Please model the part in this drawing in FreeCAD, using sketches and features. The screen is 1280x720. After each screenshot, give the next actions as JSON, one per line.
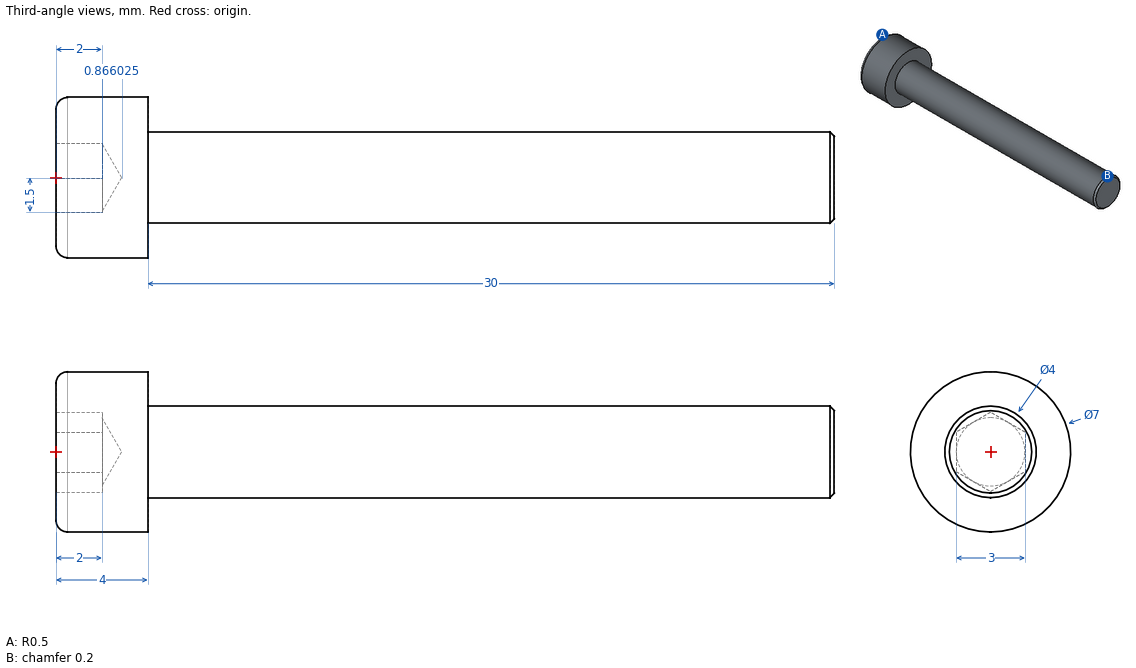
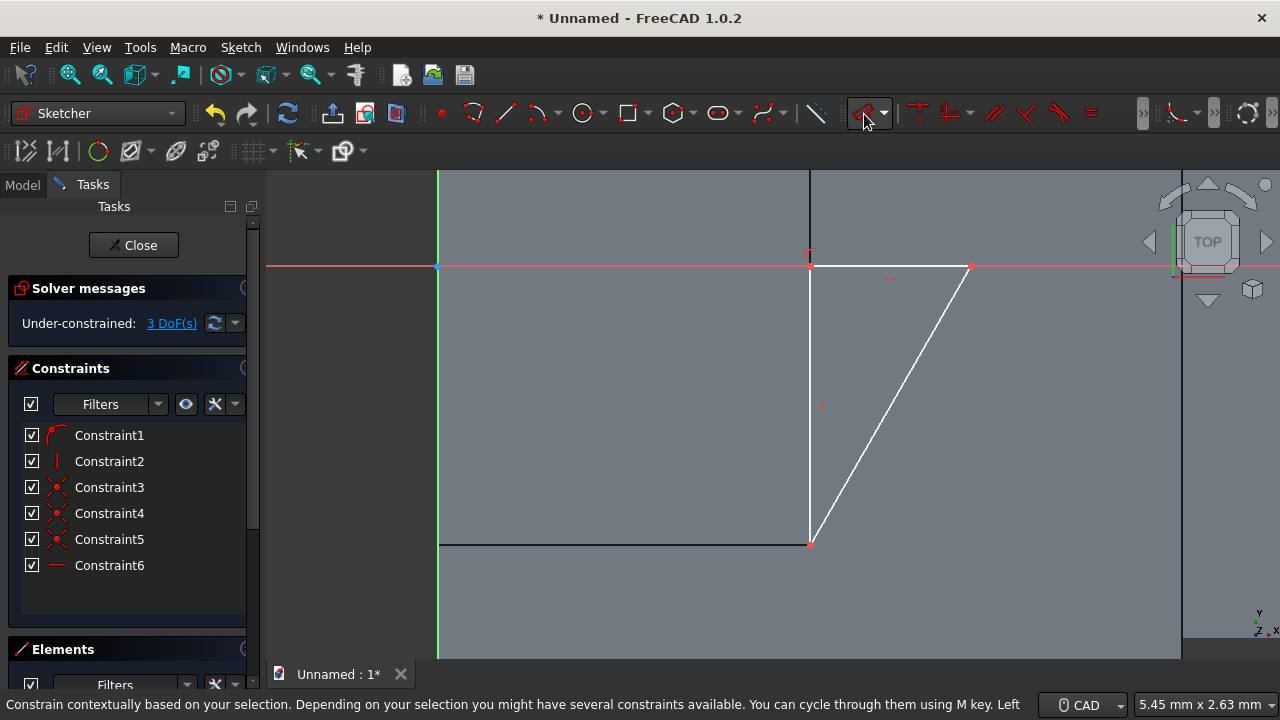
{"action": "left_click", "coordinate": [810, 266]}
{"action": "left_click", "coordinate": [624, 232]}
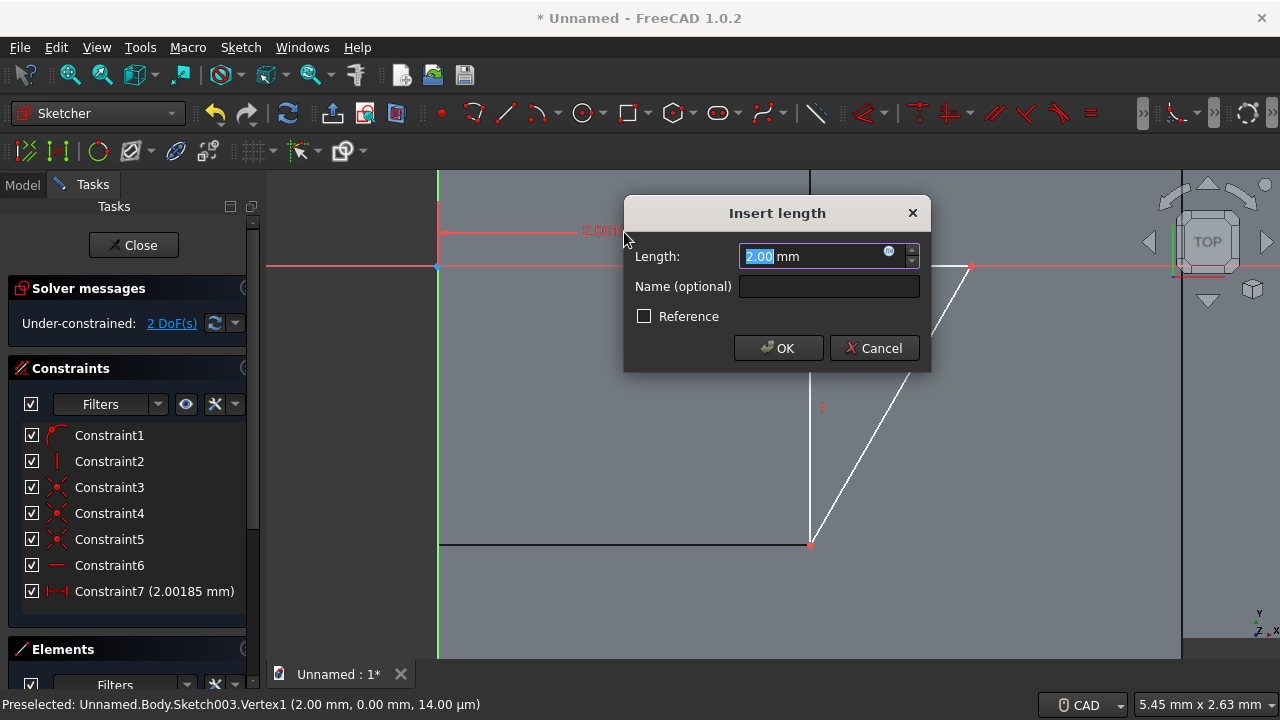
{"action": "type", "text": "2"}
{"action": "key", "text": "Return"}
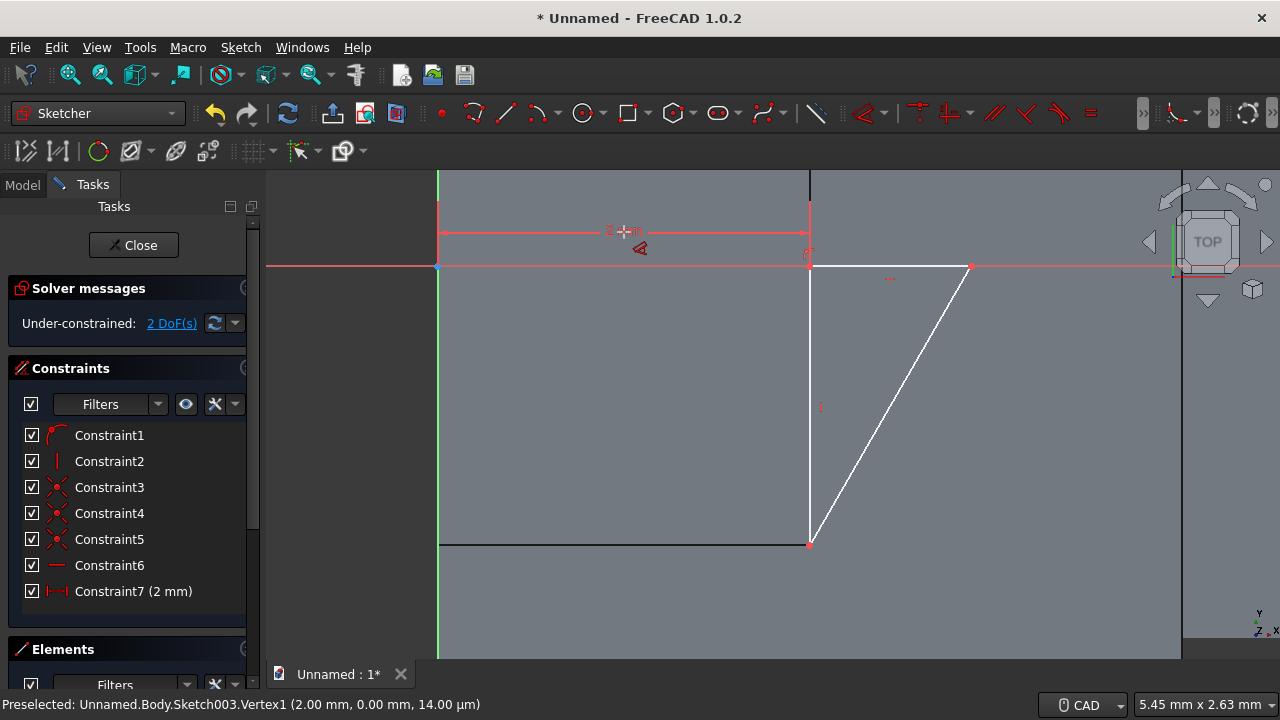
{"action": "left_click", "coordinate": [810, 350]}
{"action": "left_click", "coordinate": [844, 406]}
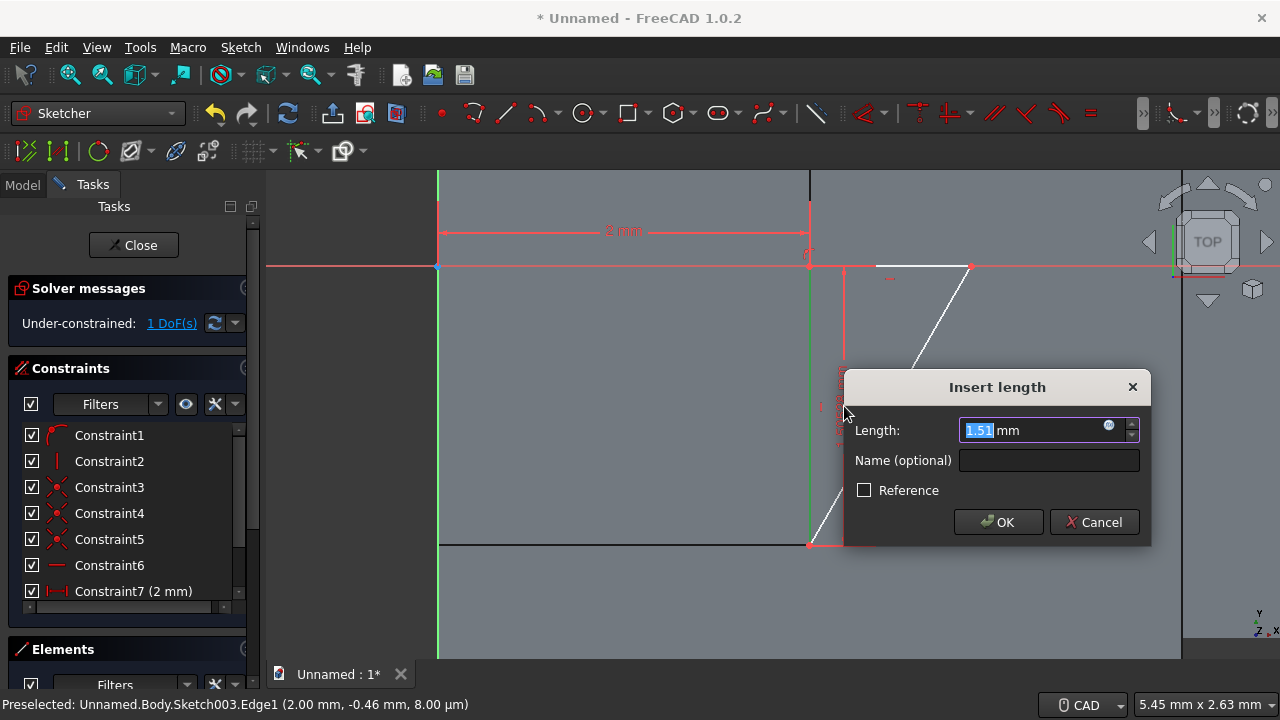
{"action": "type", "text": "1.5"}
{"action": "key", "text": "Return"}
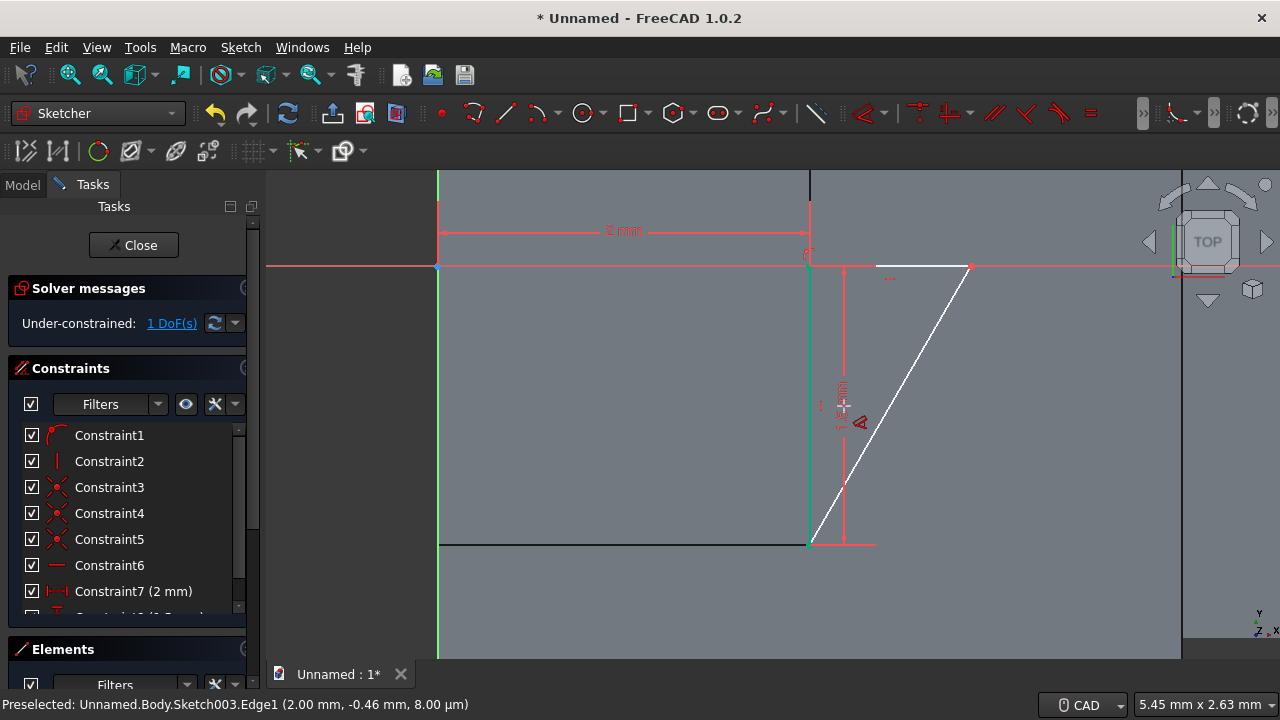
{"action": "left_click", "coordinate": [923, 266]}
{"action": "left_click", "coordinate": [890, 232]}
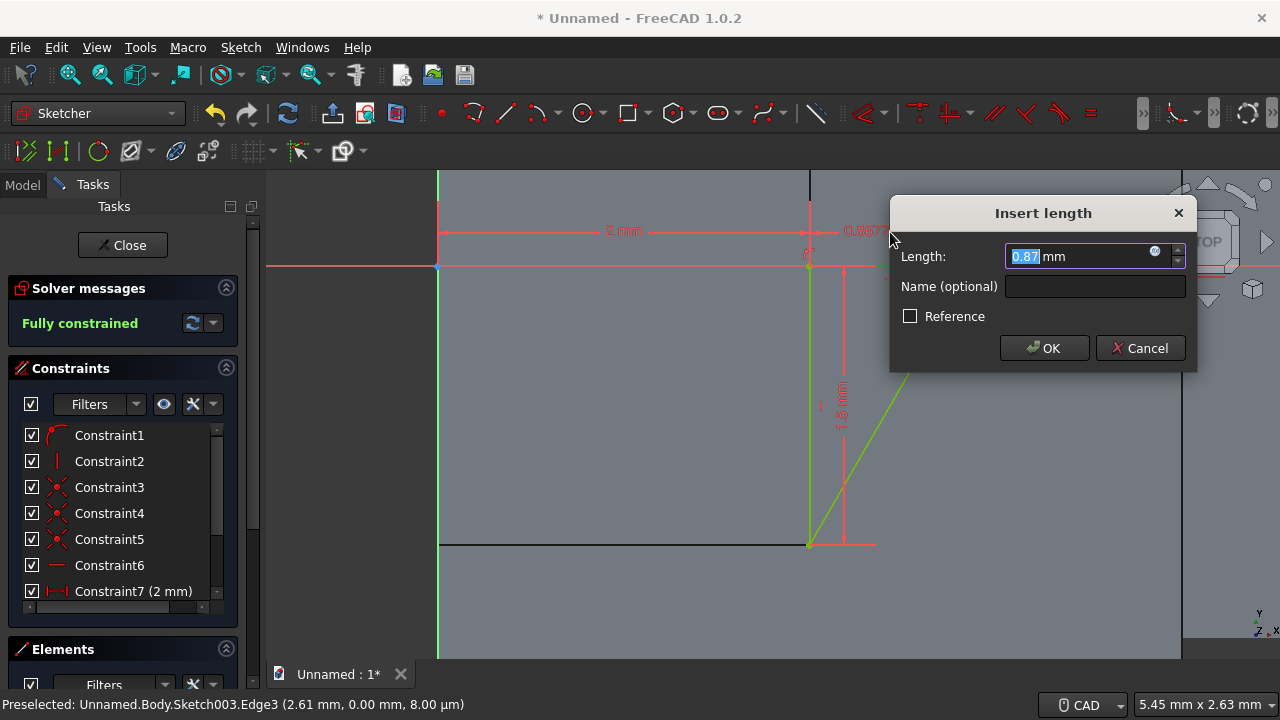
{"action": "type", "text": "0.866025"}
{"action": "key", "text": "Return"}
{"action": "key", "text": "Escape"}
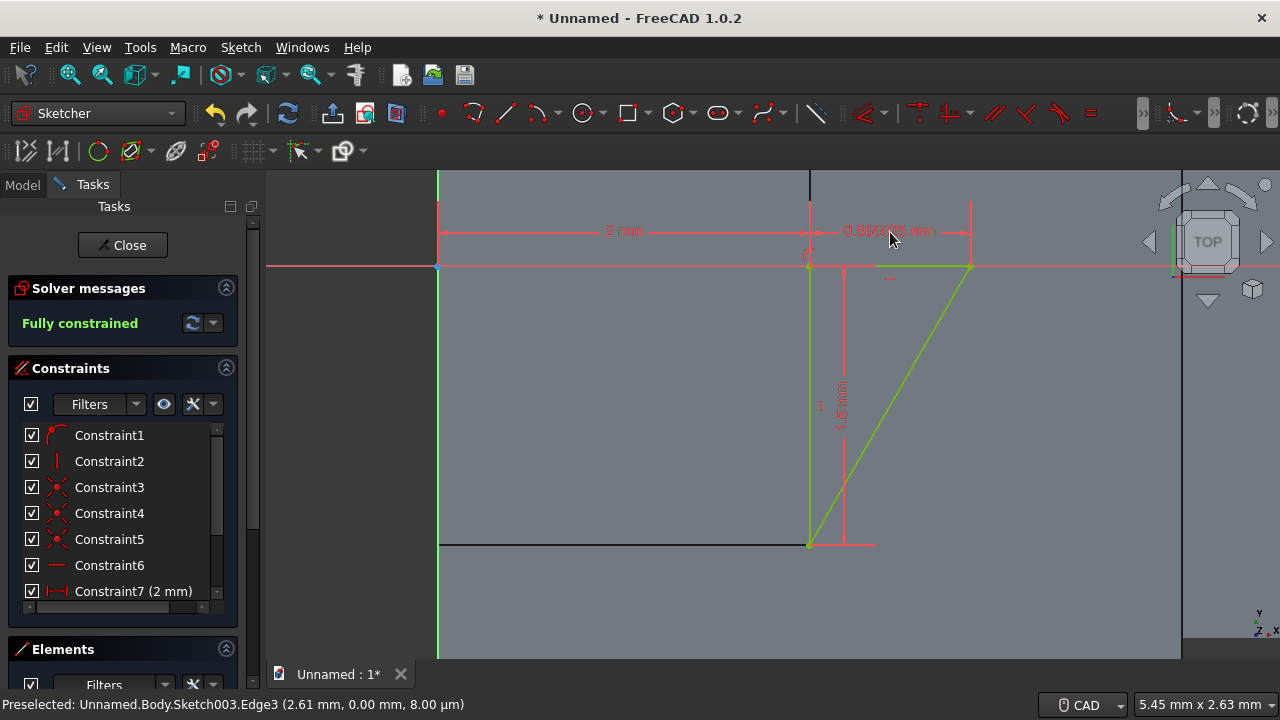
{"action": "left_click", "coordinate": [123, 245]}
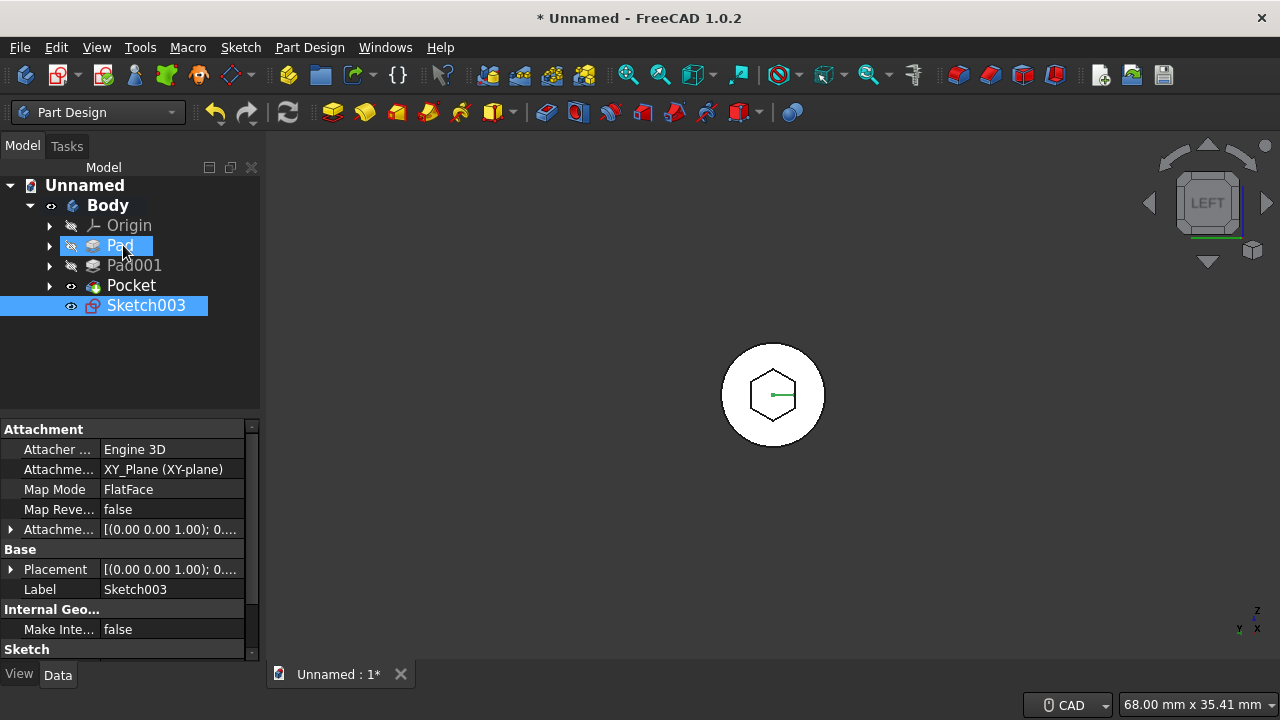
{"action": "left_click", "coordinate": [612, 112]}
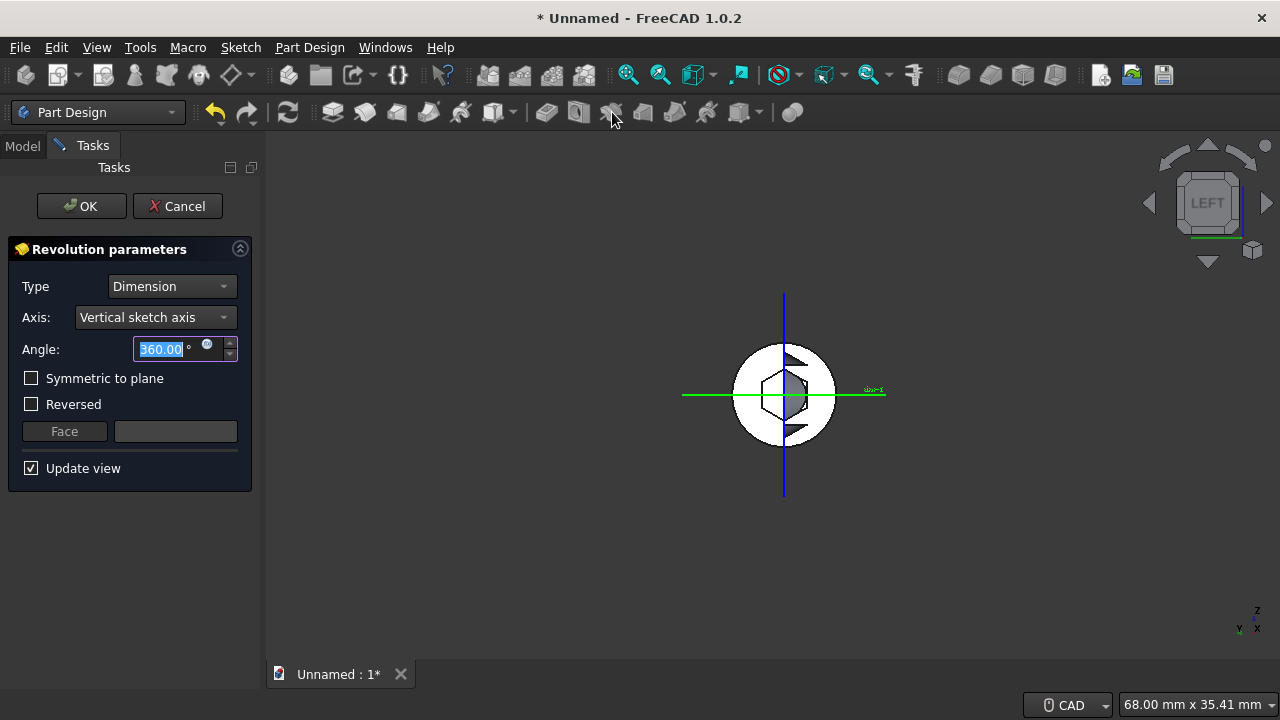
{"action": "left_click", "coordinate": [156, 318]}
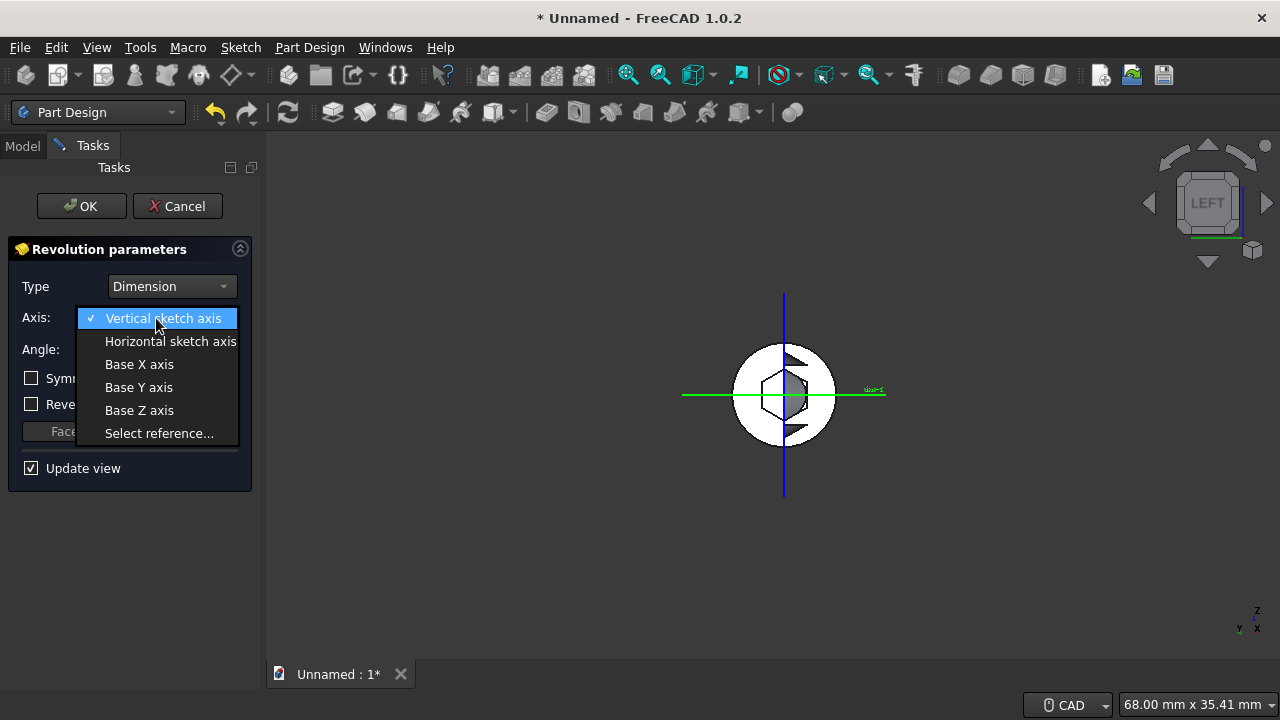
{"action": "left_click", "coordinate": [156, 342]}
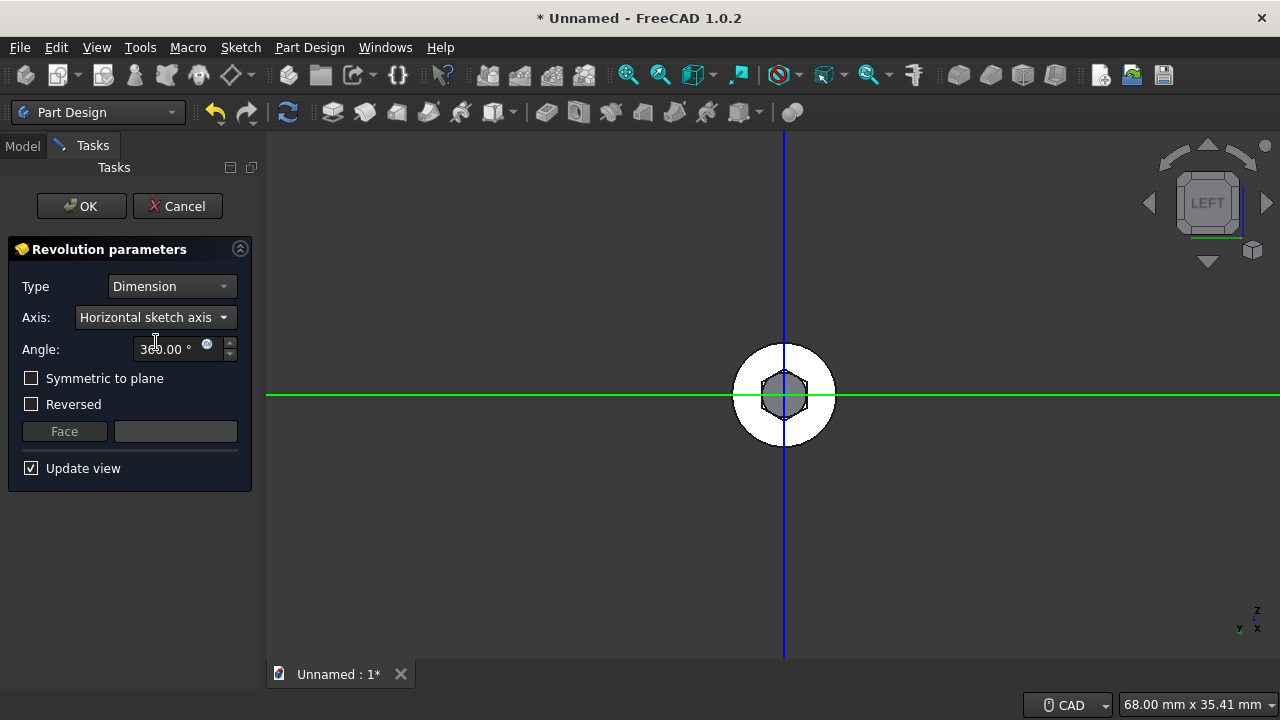
{"action": "left_click", "coordinate": [82, 206]}